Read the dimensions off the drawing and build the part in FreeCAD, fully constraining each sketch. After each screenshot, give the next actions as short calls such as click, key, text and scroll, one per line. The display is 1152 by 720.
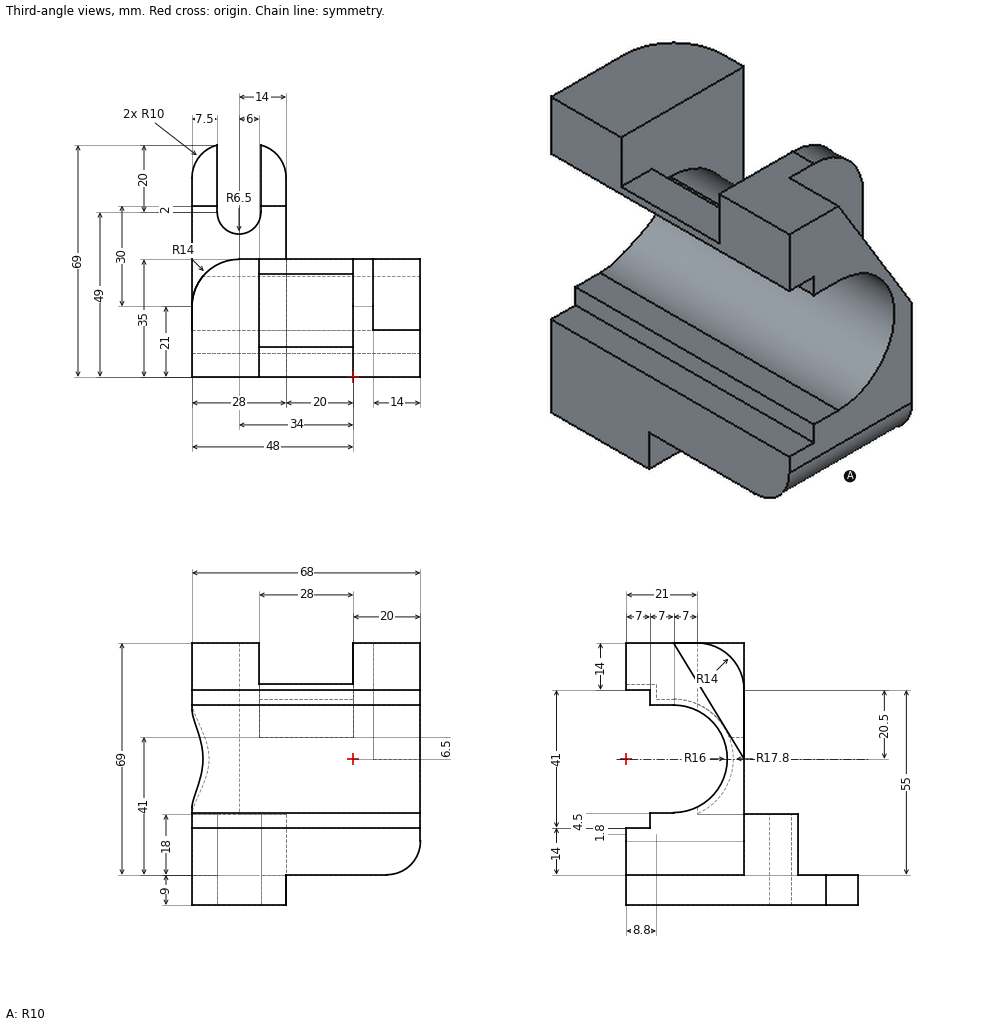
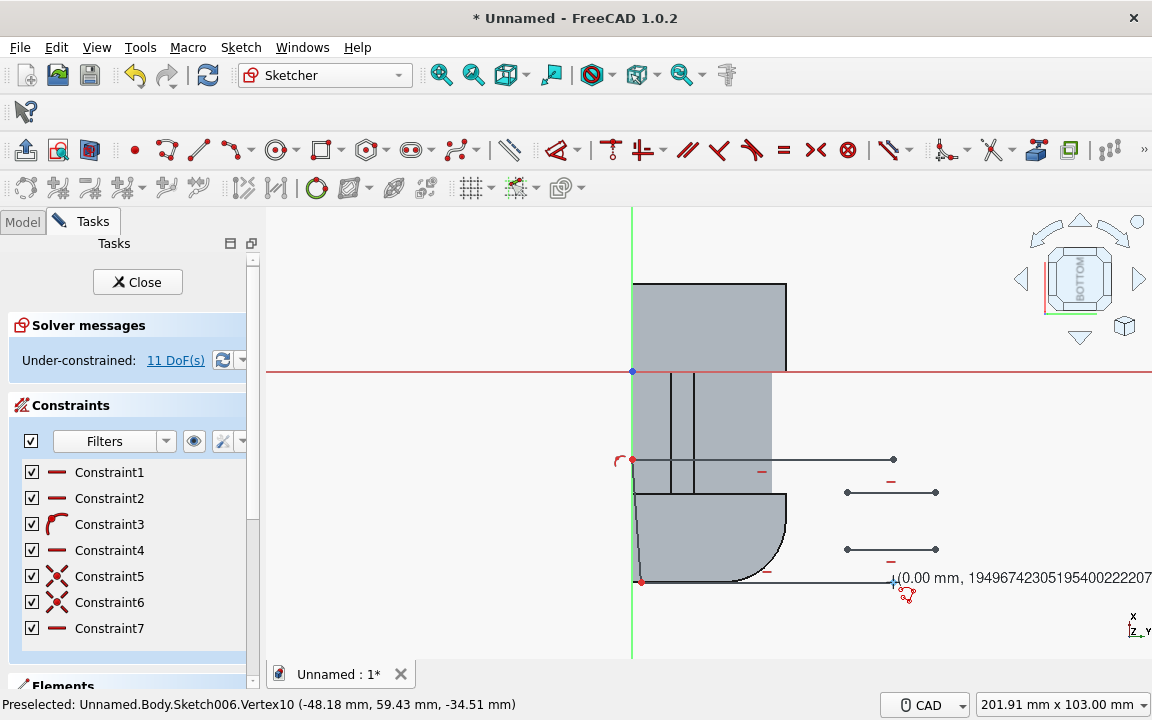
key(g)
key(3)
key(a)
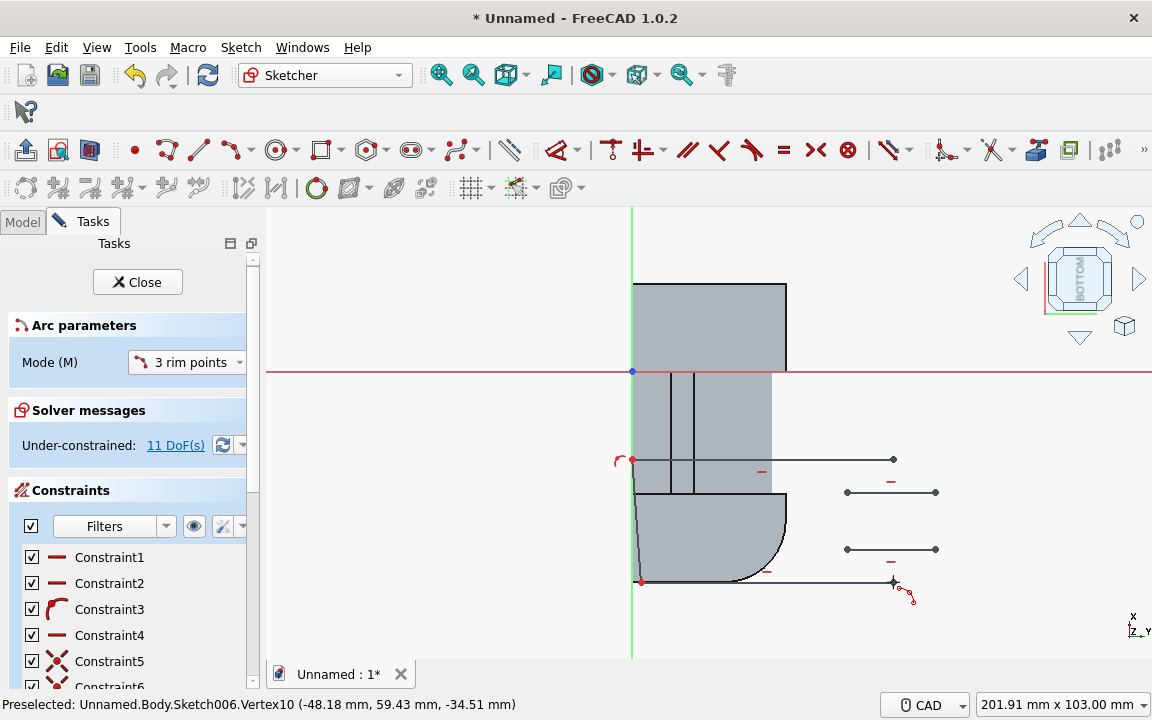
click(847, 550)
click(847, 493)
click(819, 521)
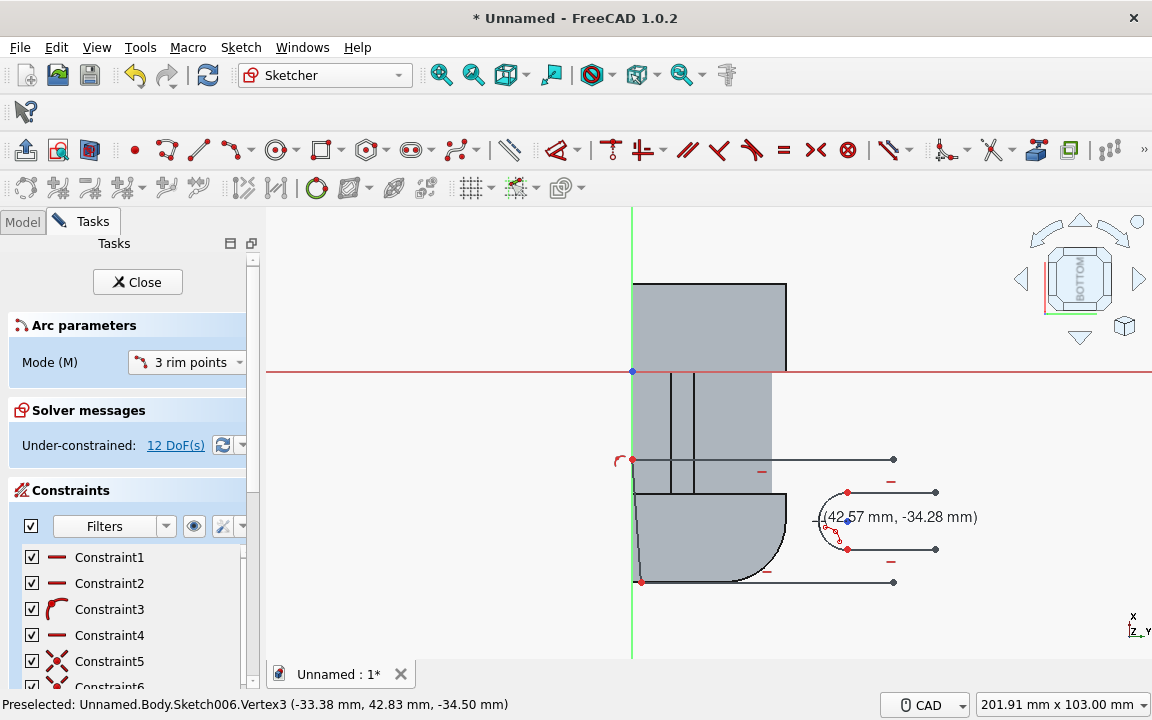
click(935, 493)
click(893, 460)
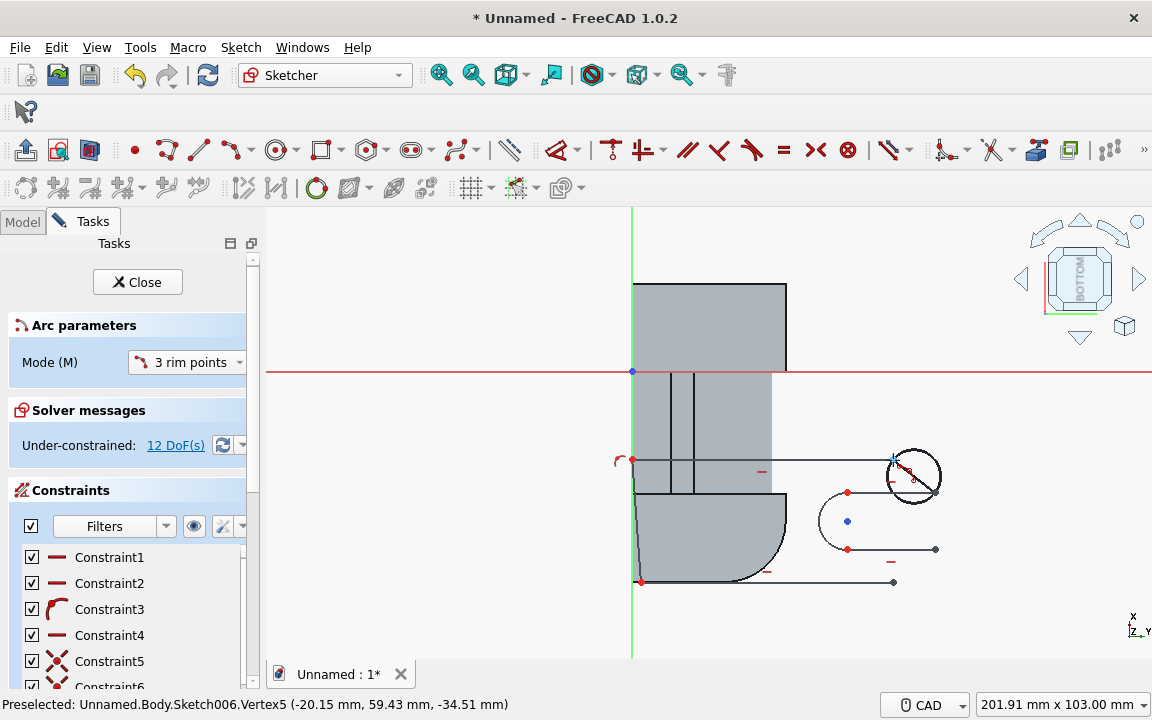
scroll(919, 469, up, 3)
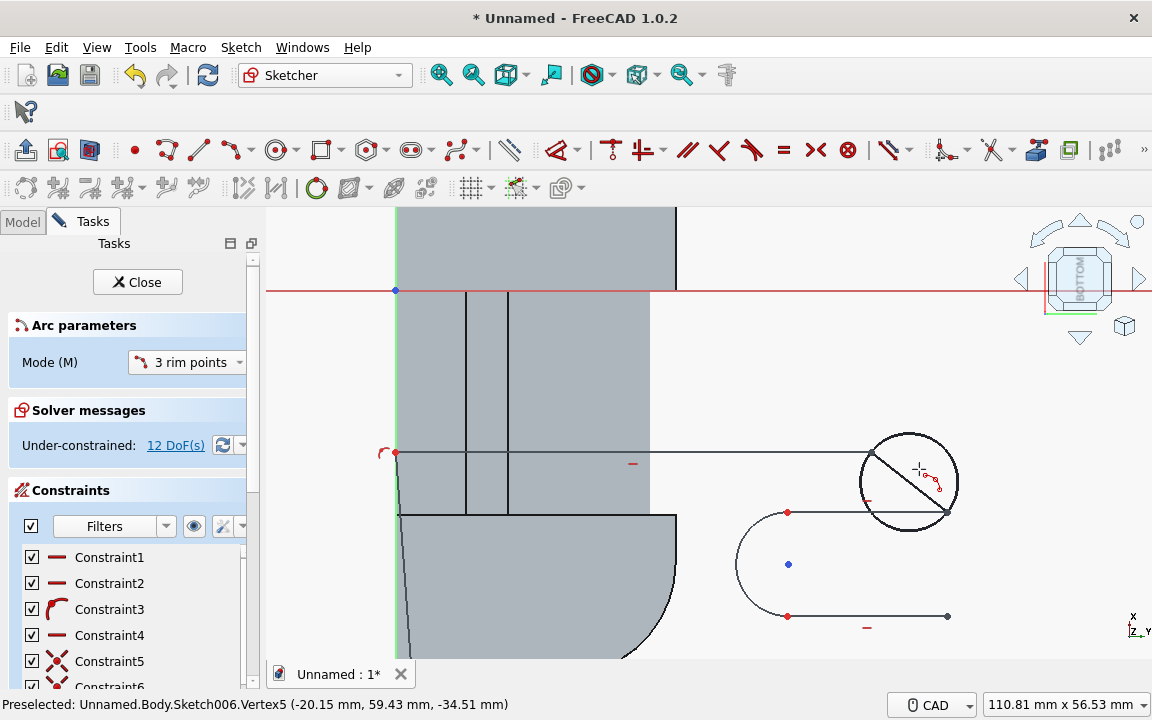
click(919, 468)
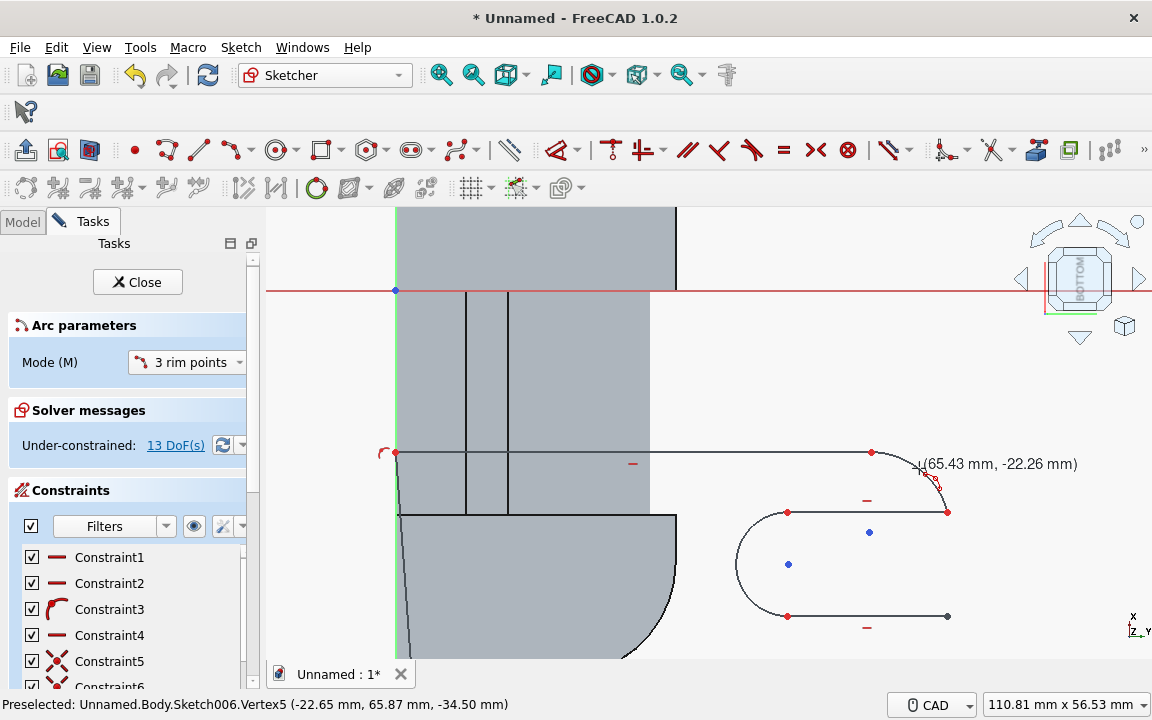
scroll(577, 332, down, 2)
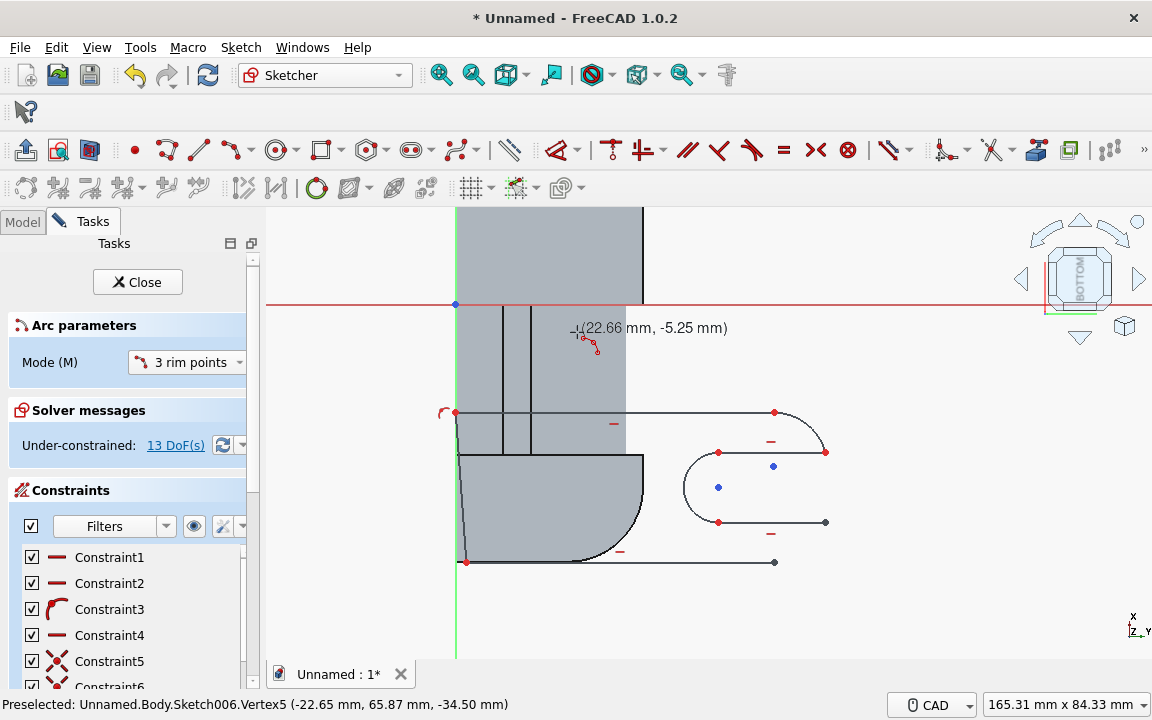
click(774, 563)
click(826, 523)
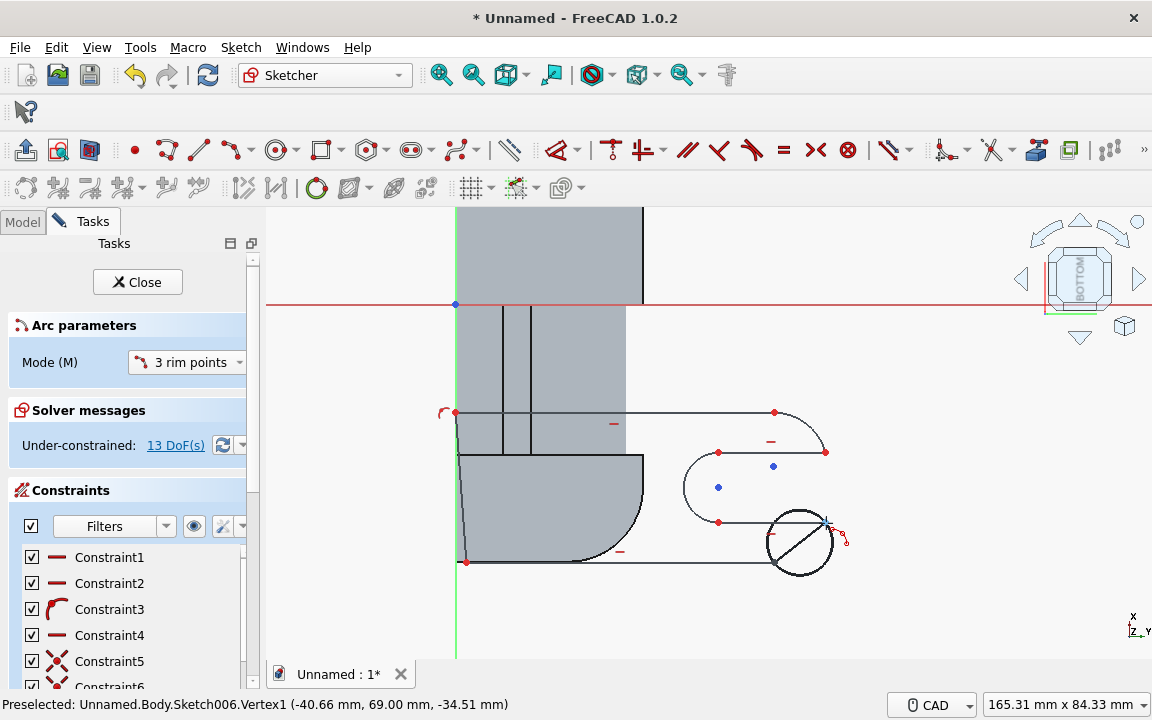
scroll(806, 551, up, 2)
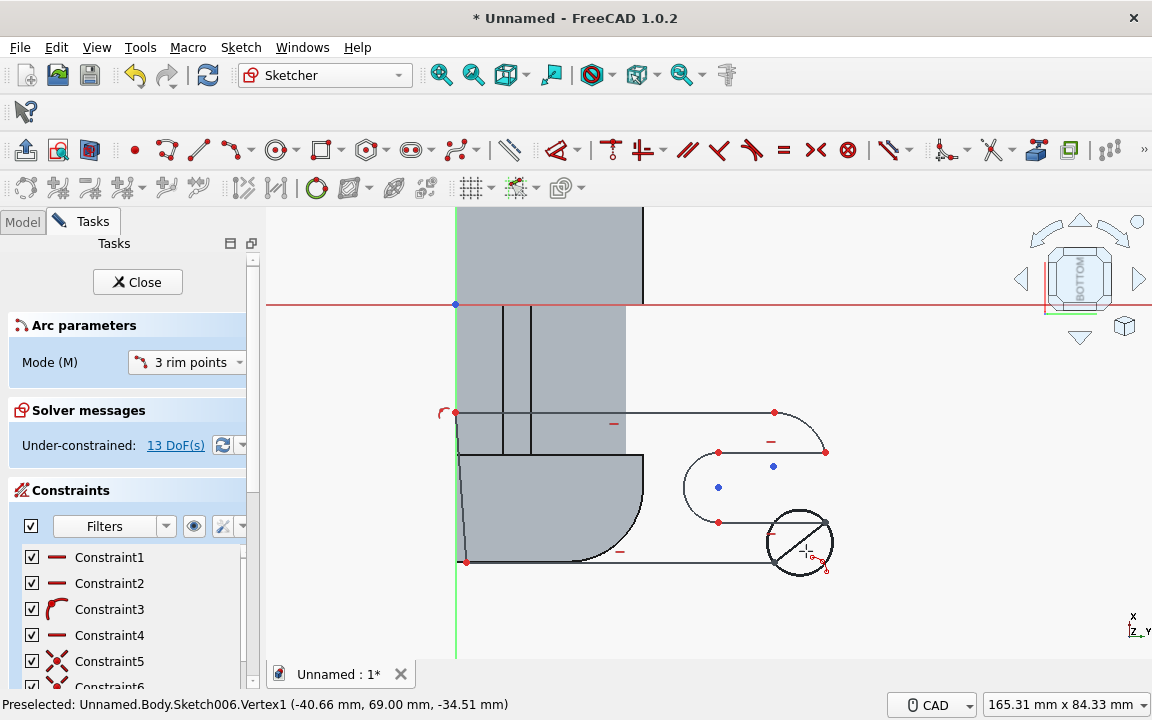
click(806, 550)
key(Escape)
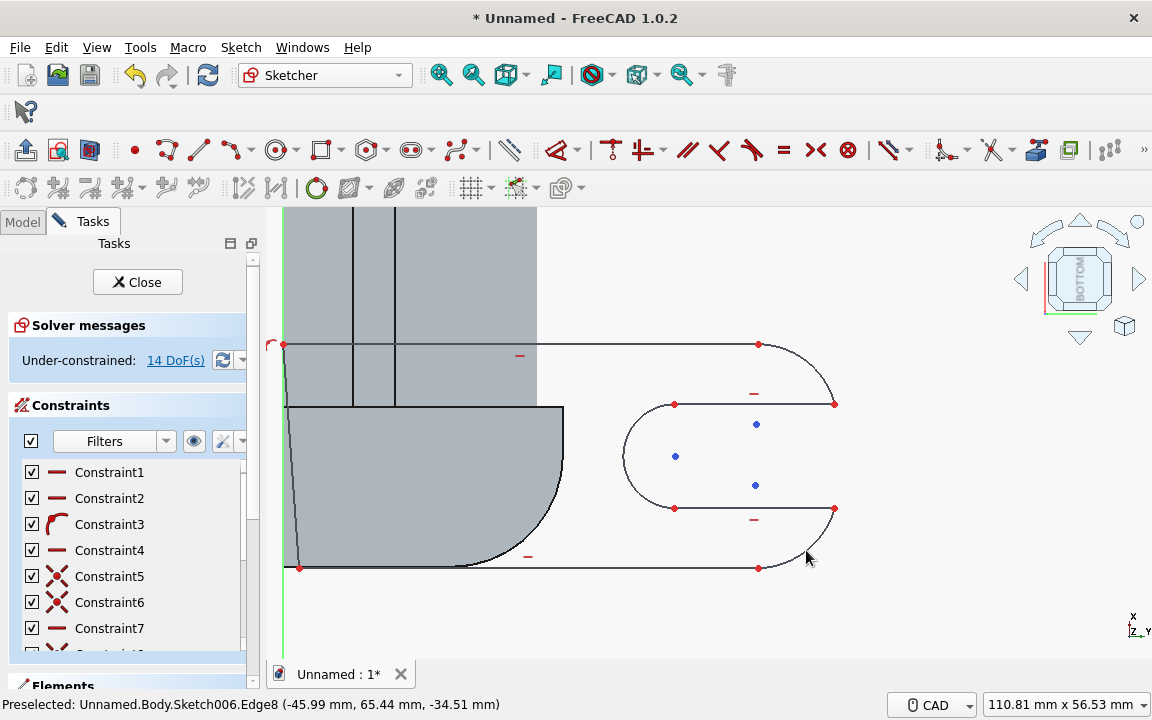
click(787, 508)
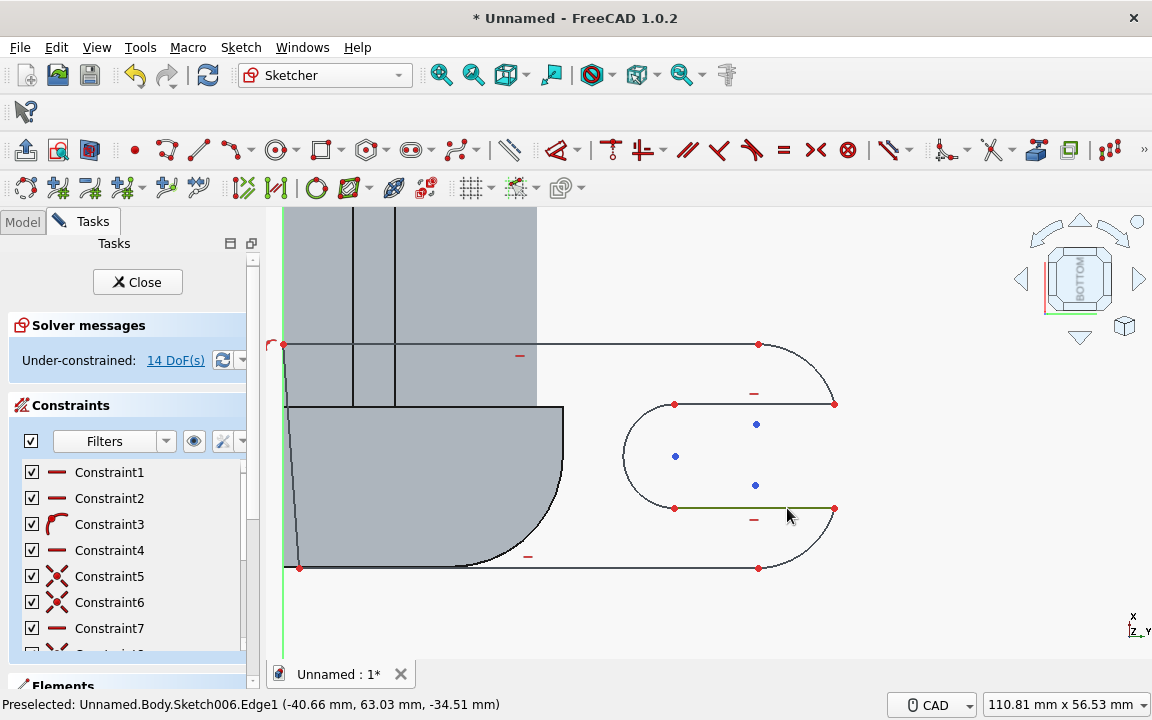
click(633, 426)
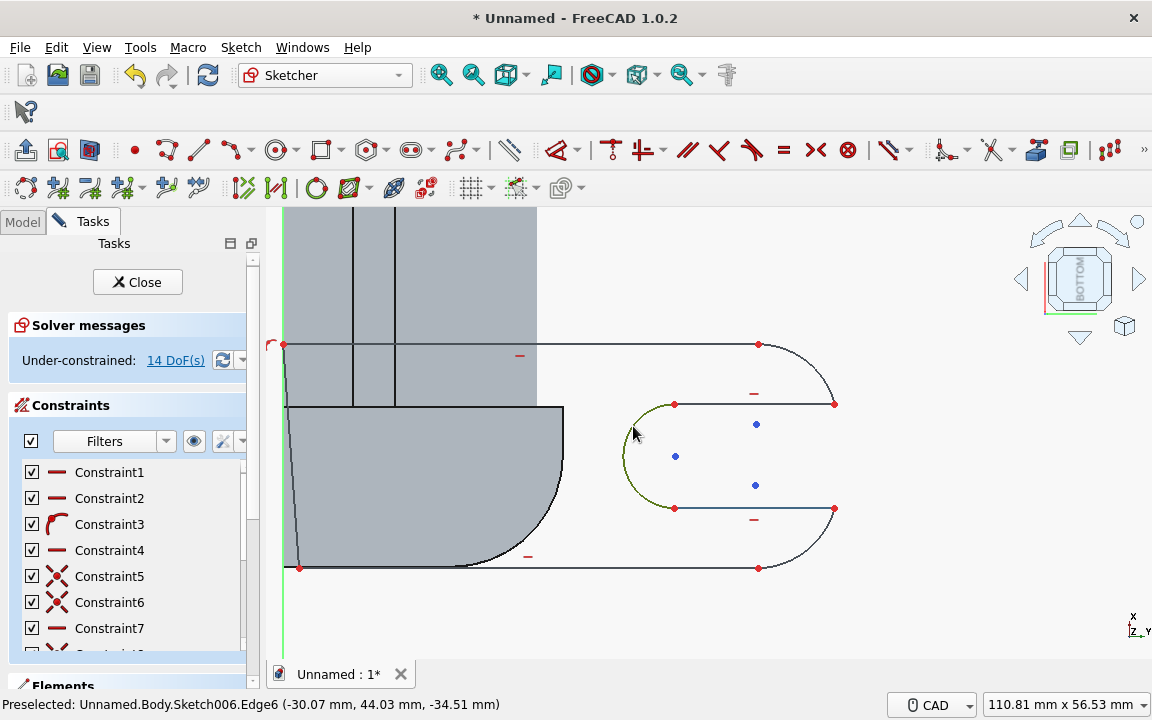
key(t)